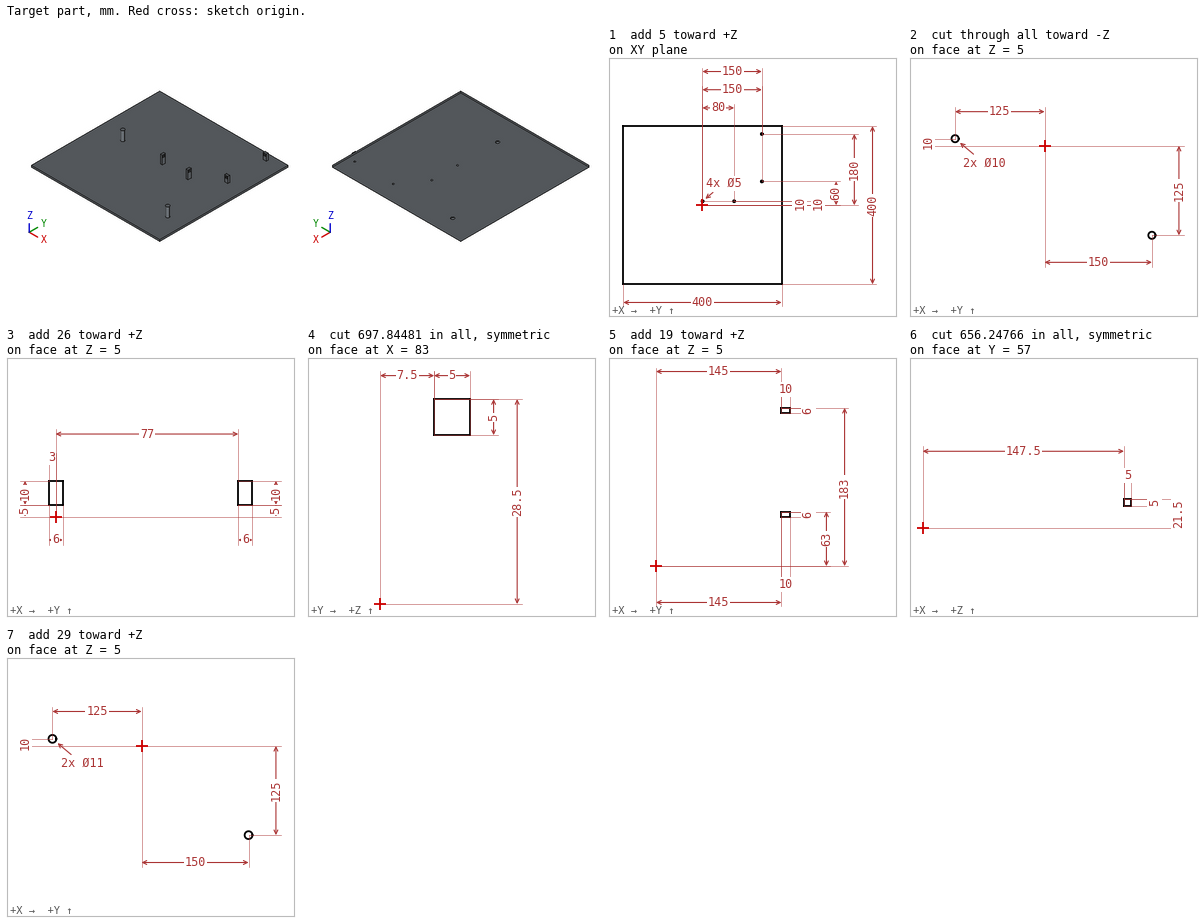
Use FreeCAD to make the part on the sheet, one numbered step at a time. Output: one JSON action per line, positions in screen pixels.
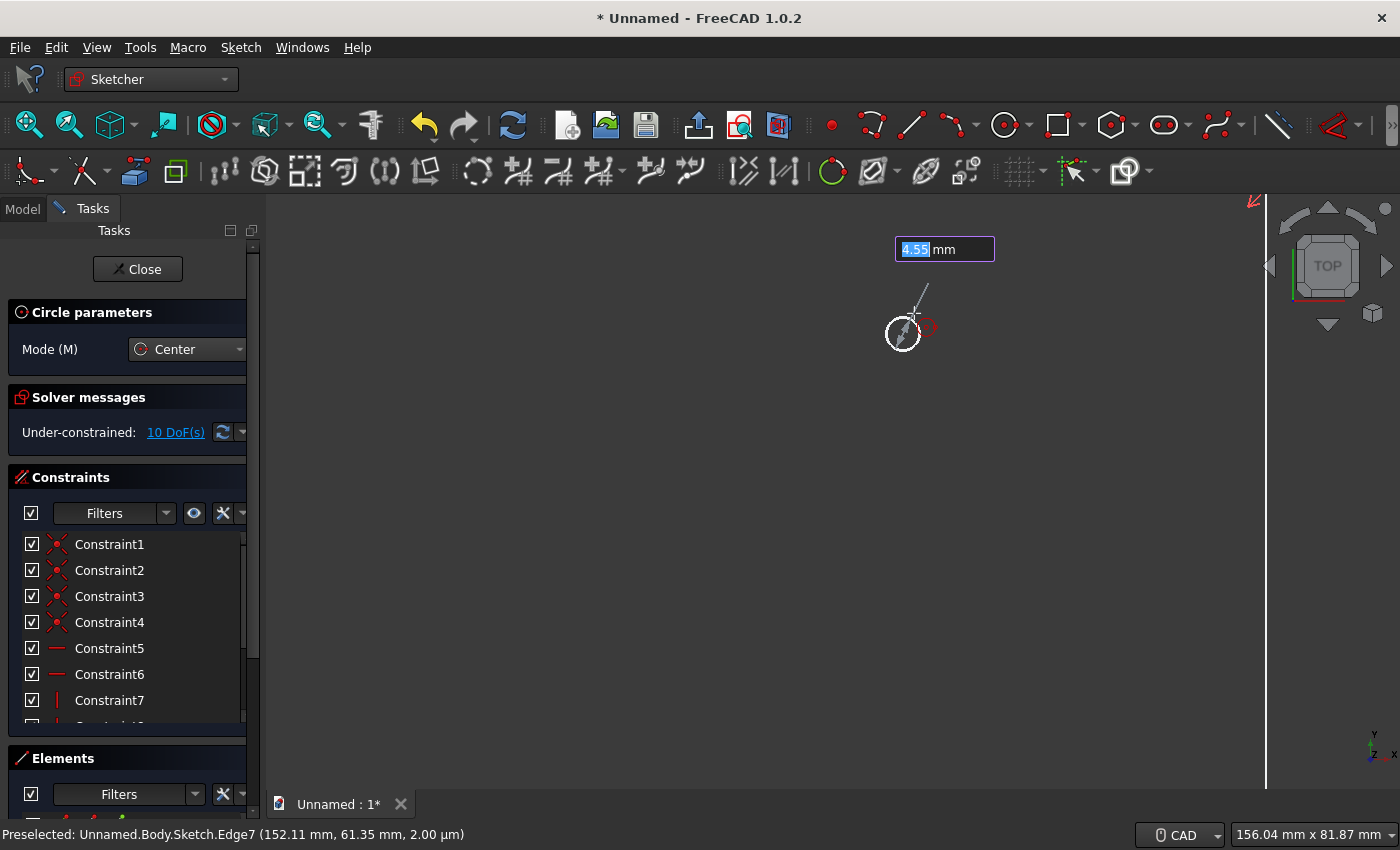
{"action": "left_click", "coordinate": [913, 312]}
{"action": "key", "text": "Escape"}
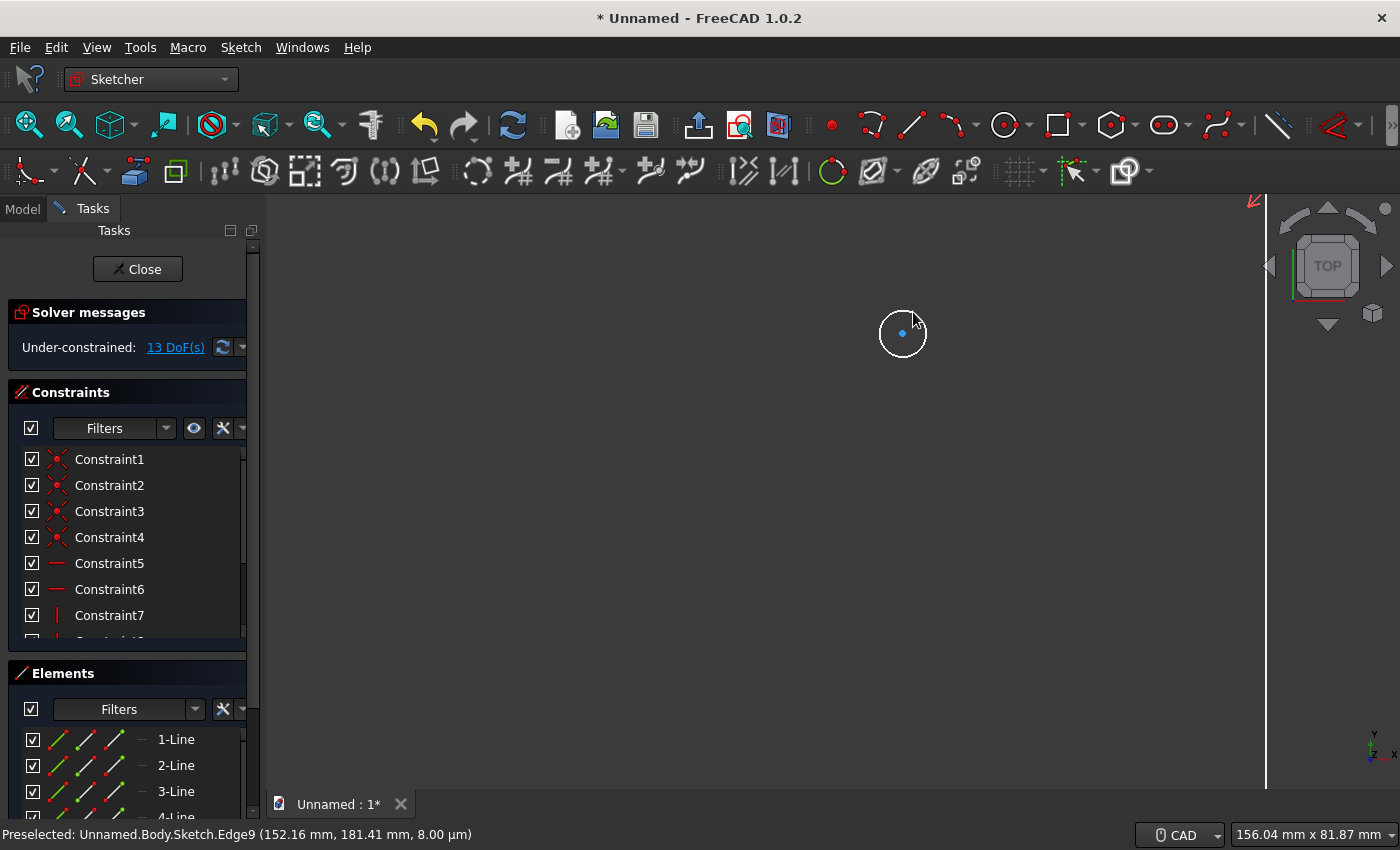
{"action": "scroll", "coordinate": [914, 313], "scroll_direction": "down", "scroll_amount": 10}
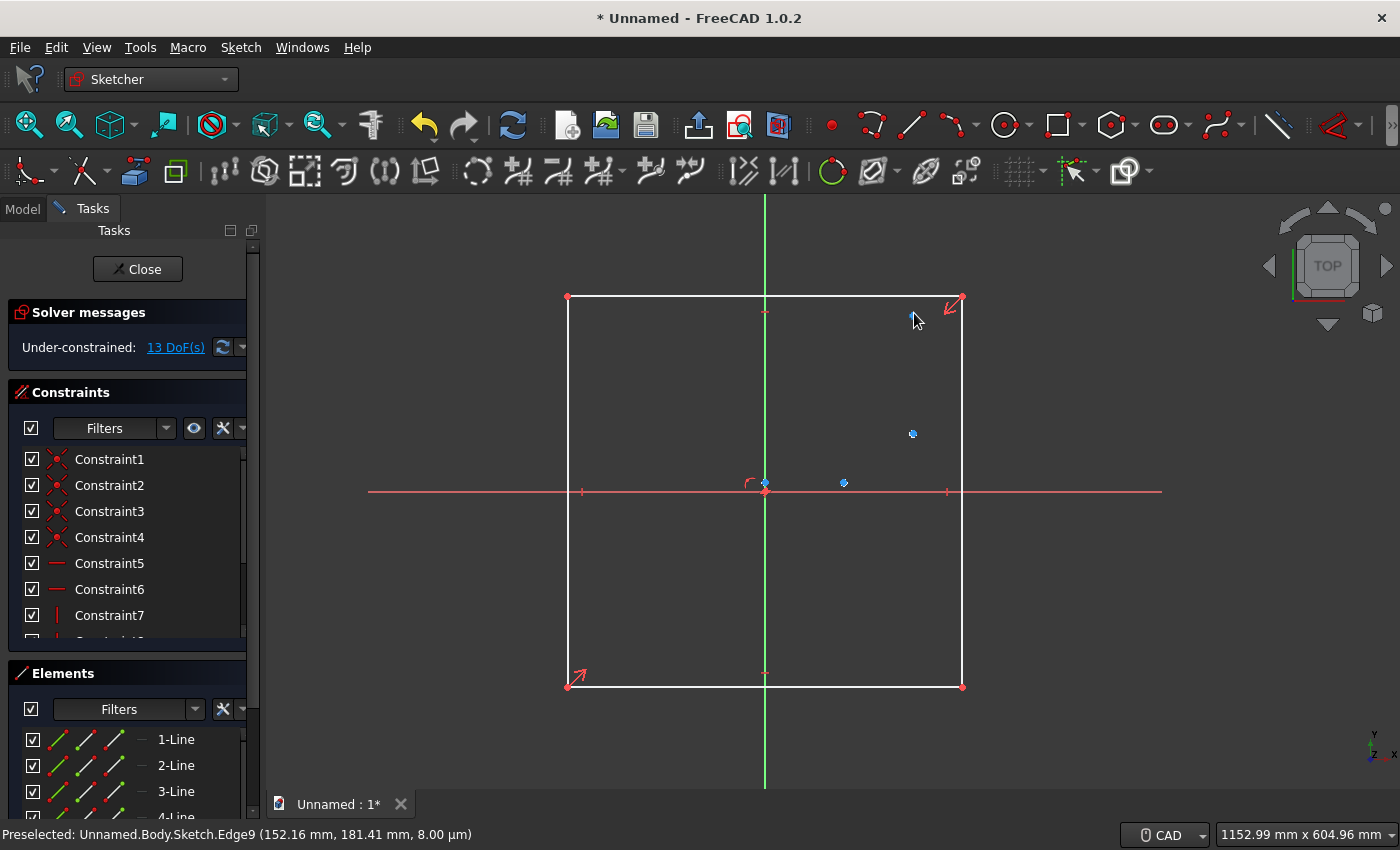
{"action": "scroll", "coordinate": [767, 481], "scroll_direction": "up", "scroll_amount": 10}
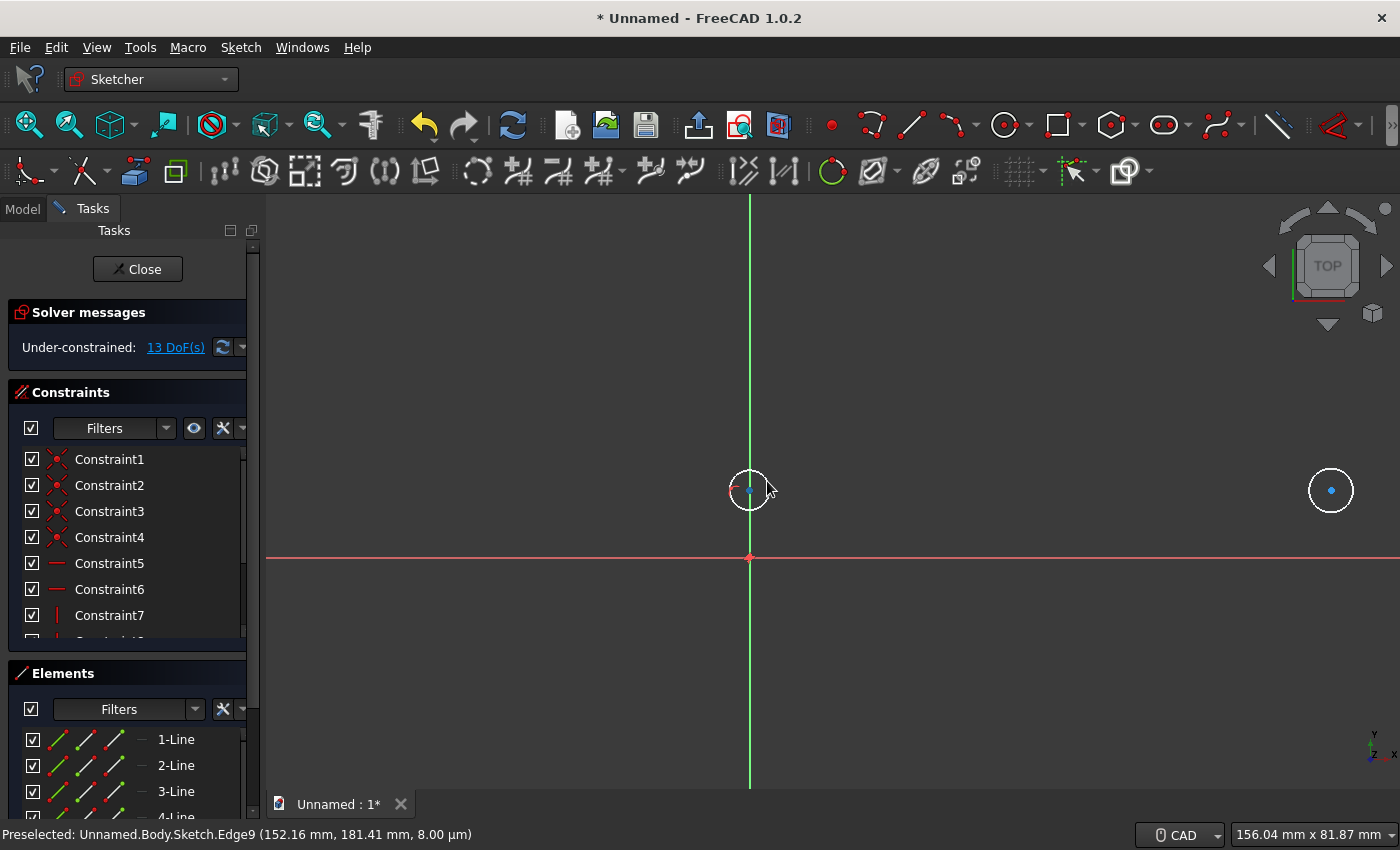
{"action": "left_click", "coordinate": [764, 476]}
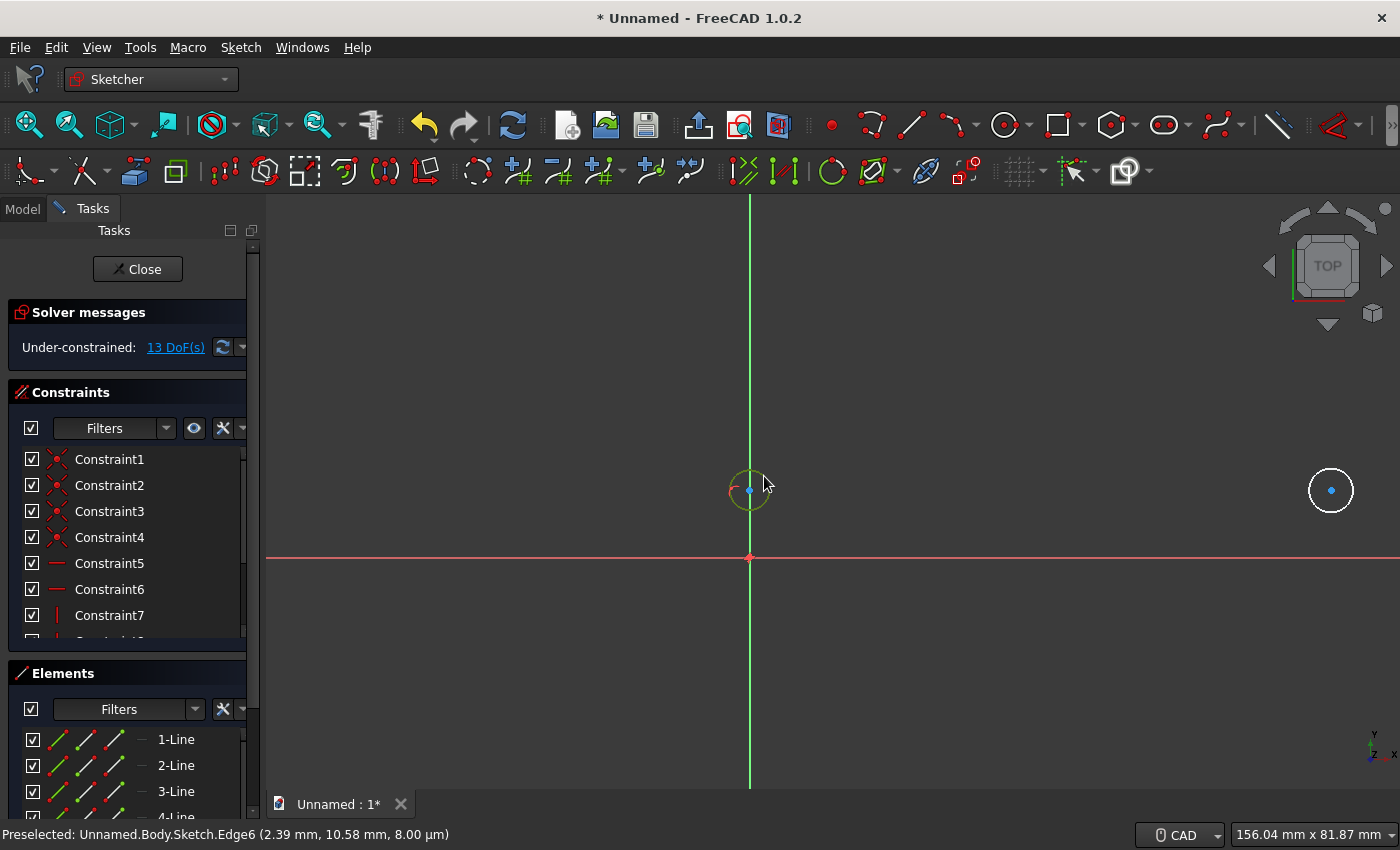
{"action": "scroll", "coordinate": [767, 481], "scroll_direction": "down", "scroll_amount": 10}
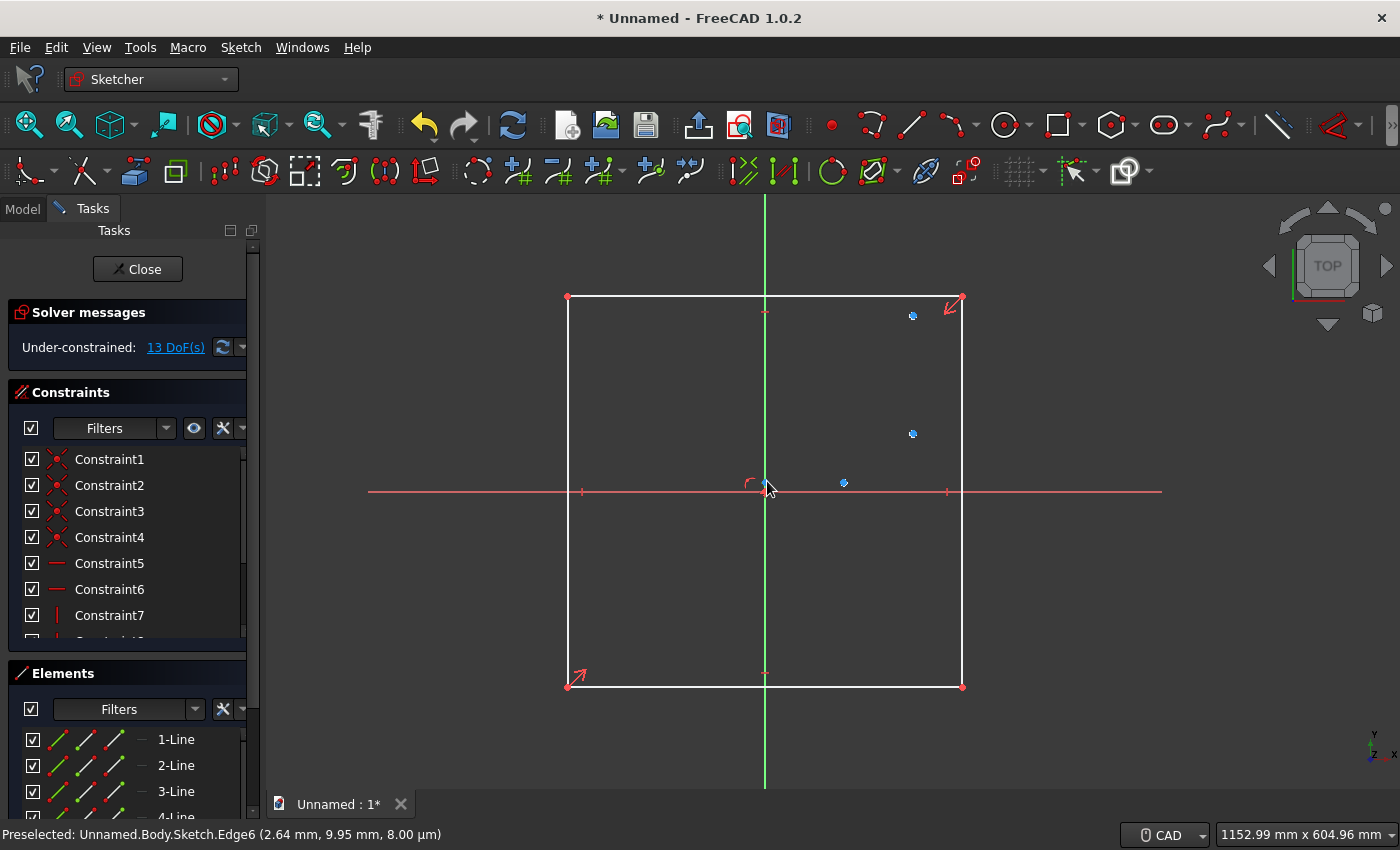
{"action": "scroll", "coordinate": [846, 481], "scroll_direction": "up", "scroll_amount": 8}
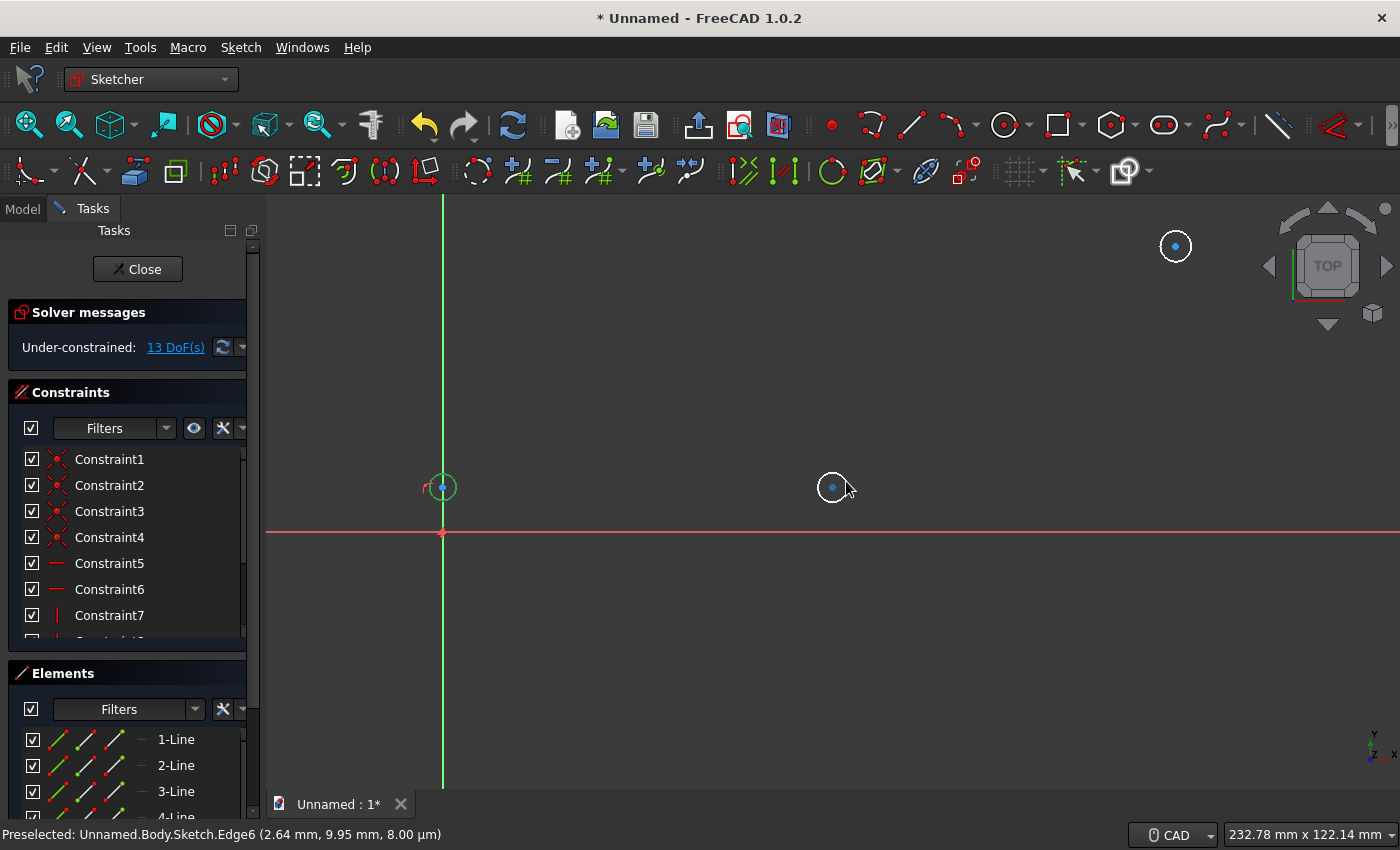
{"action": "left_click", "coordinate": [843, 477]}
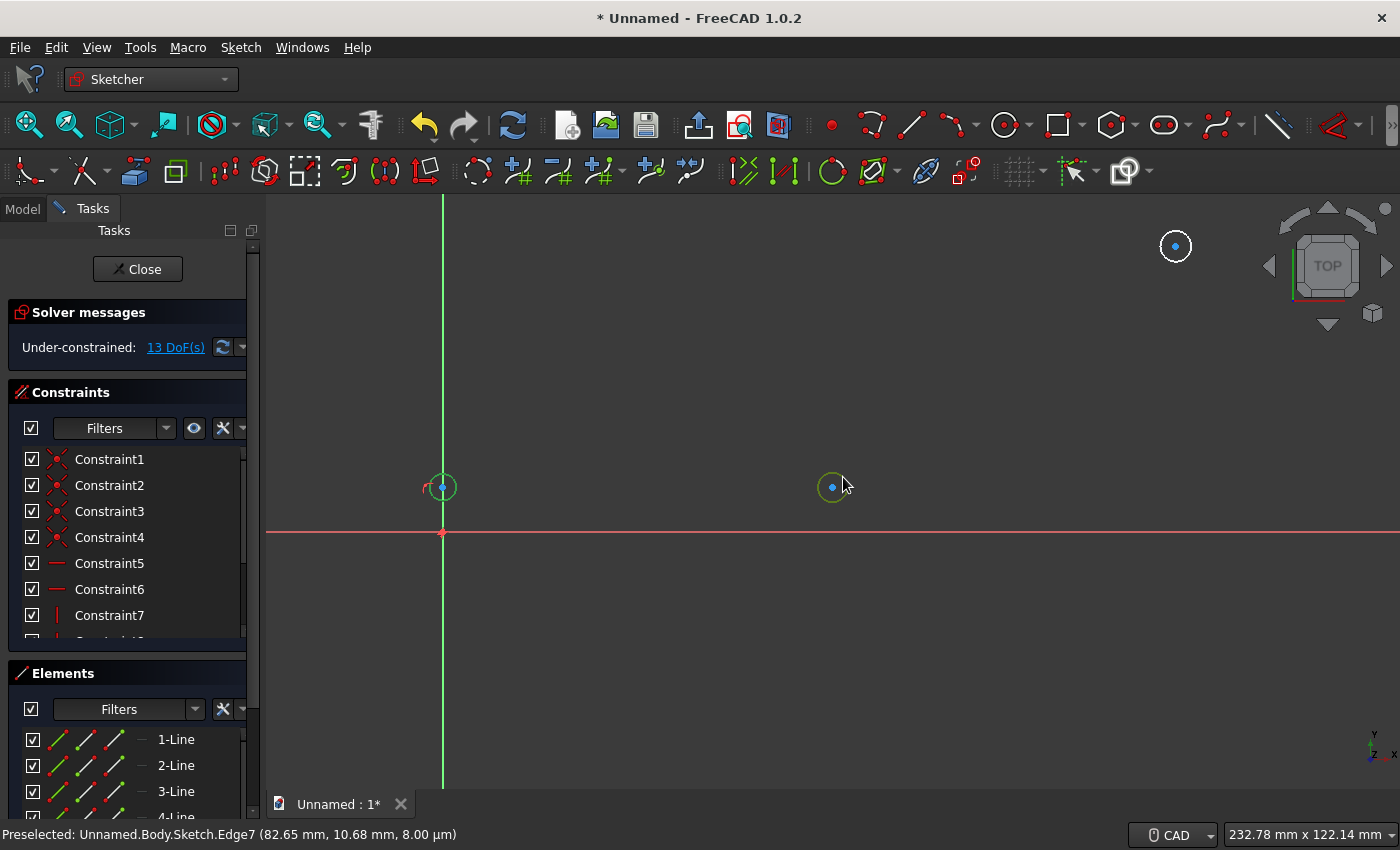
{"action": "left_click", "coordinate": [1187, 235]}